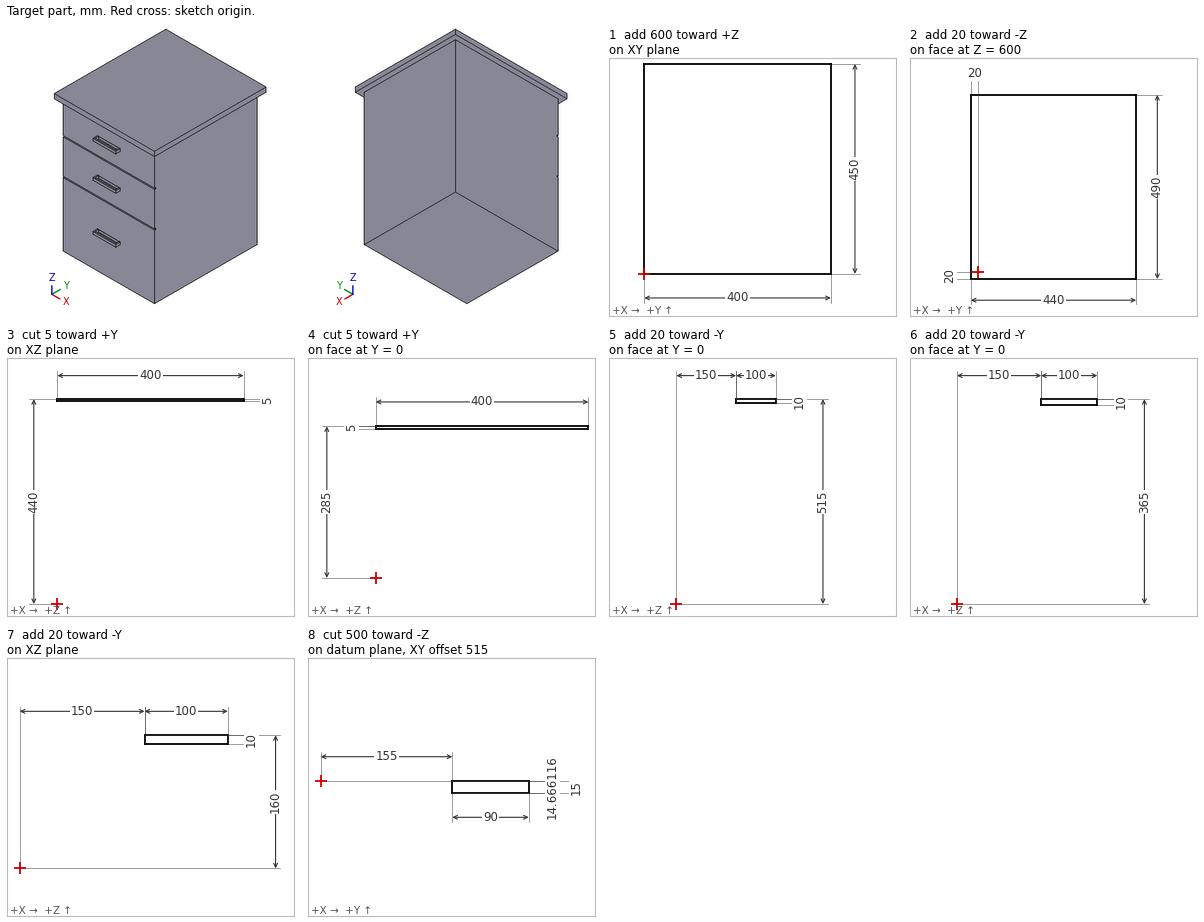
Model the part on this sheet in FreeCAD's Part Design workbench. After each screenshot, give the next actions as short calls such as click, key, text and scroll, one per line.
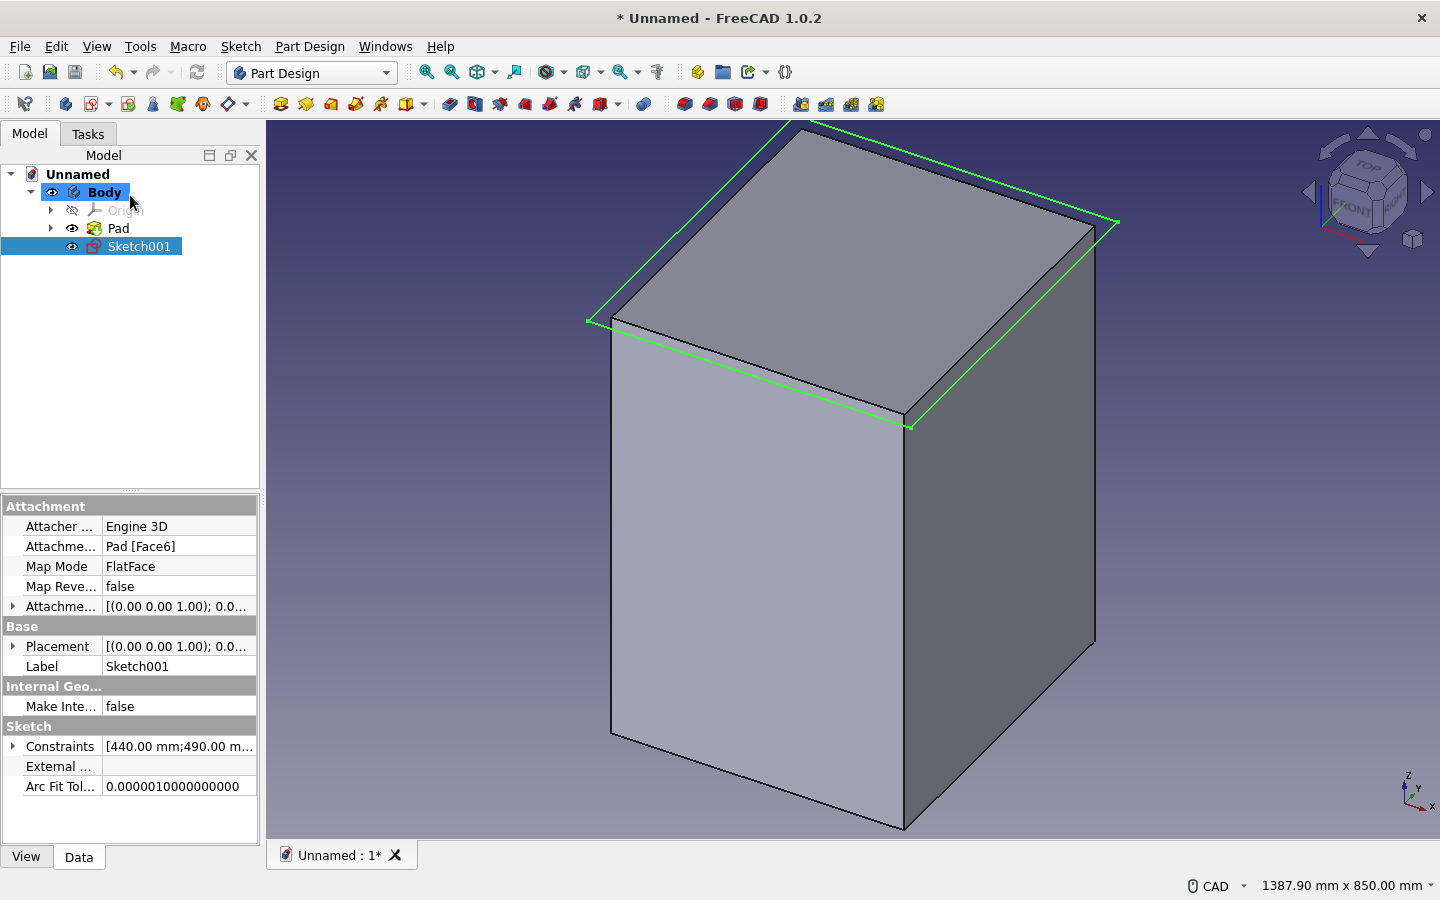
click(281, 104)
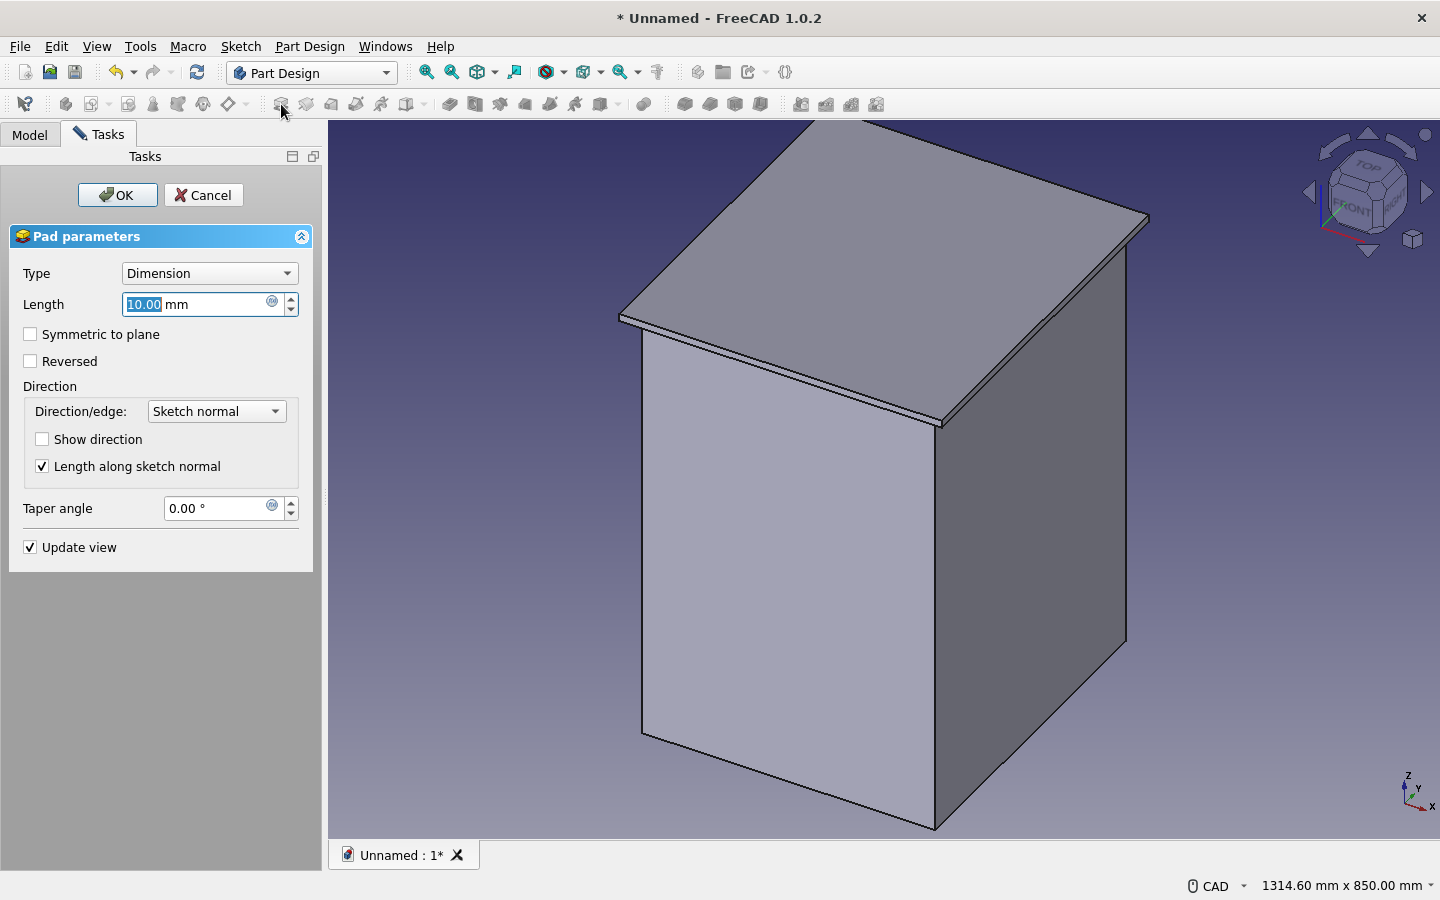
text(20)
key(Tab)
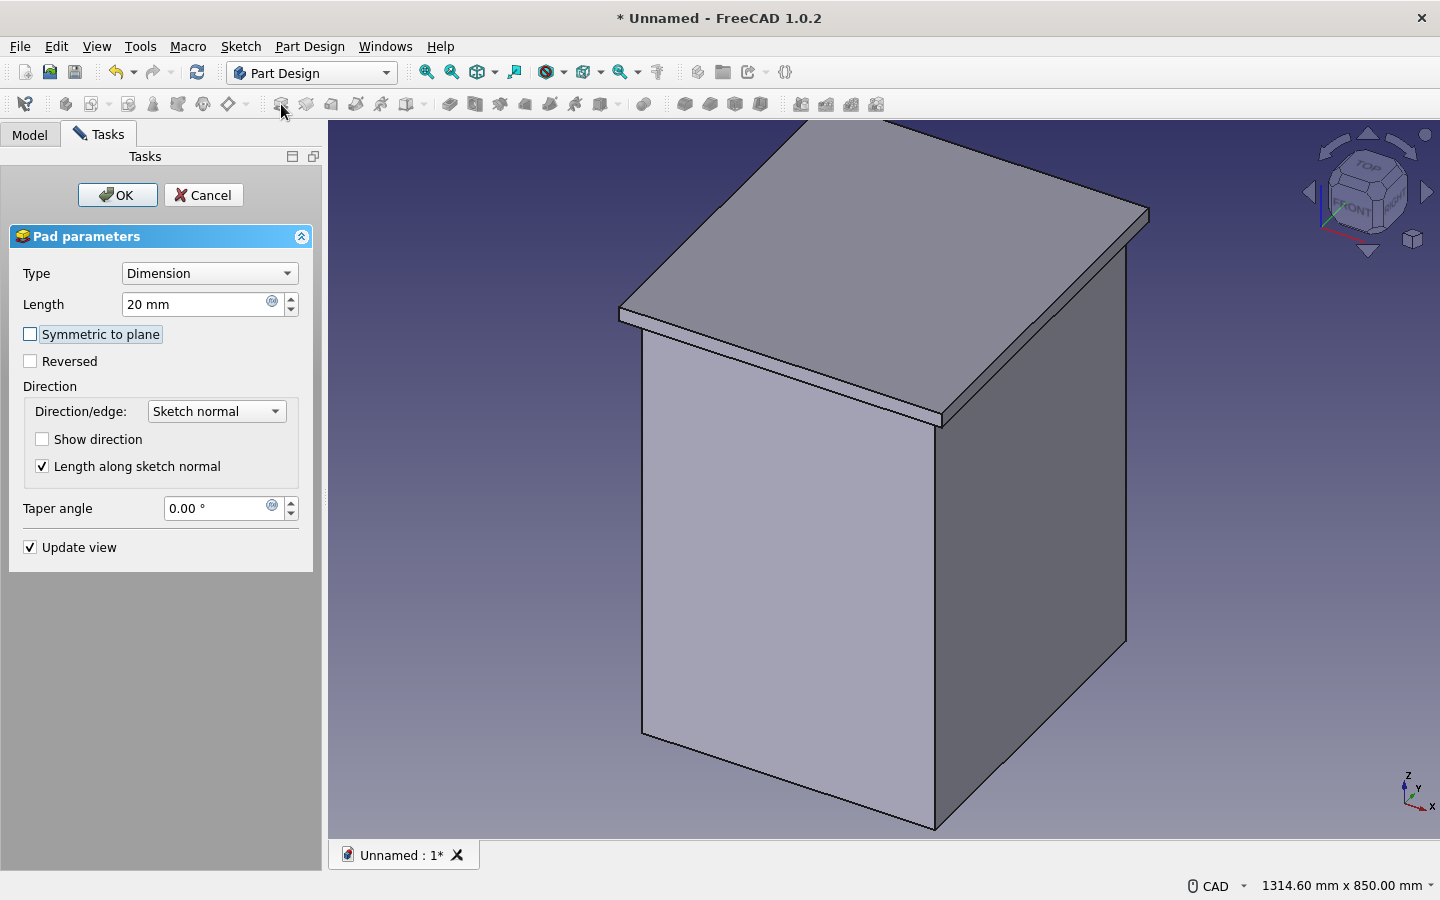
click(31, 361)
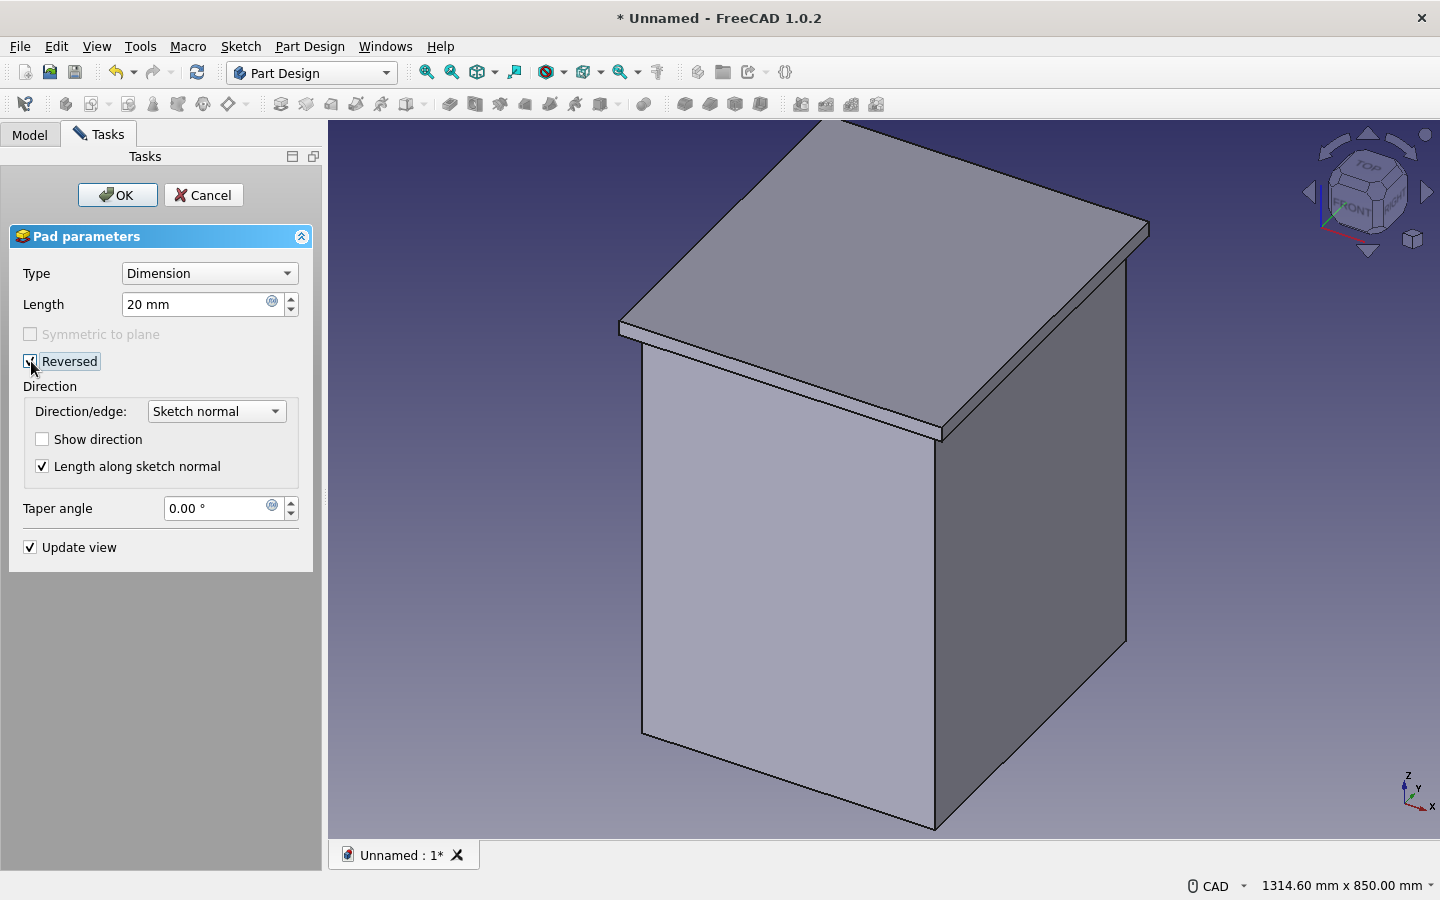
click(118, 195)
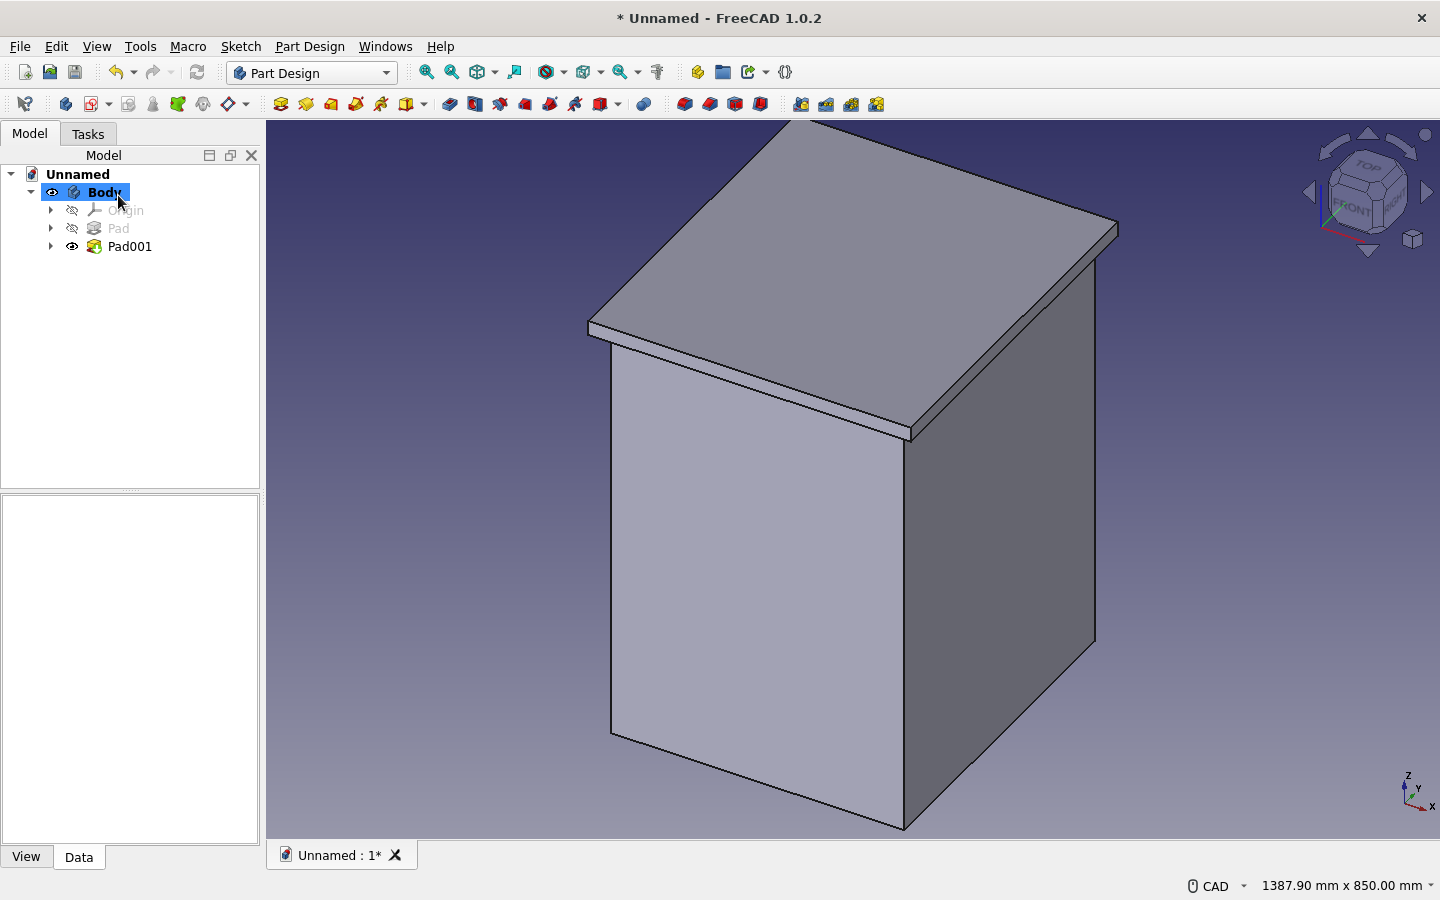
click(427, 72)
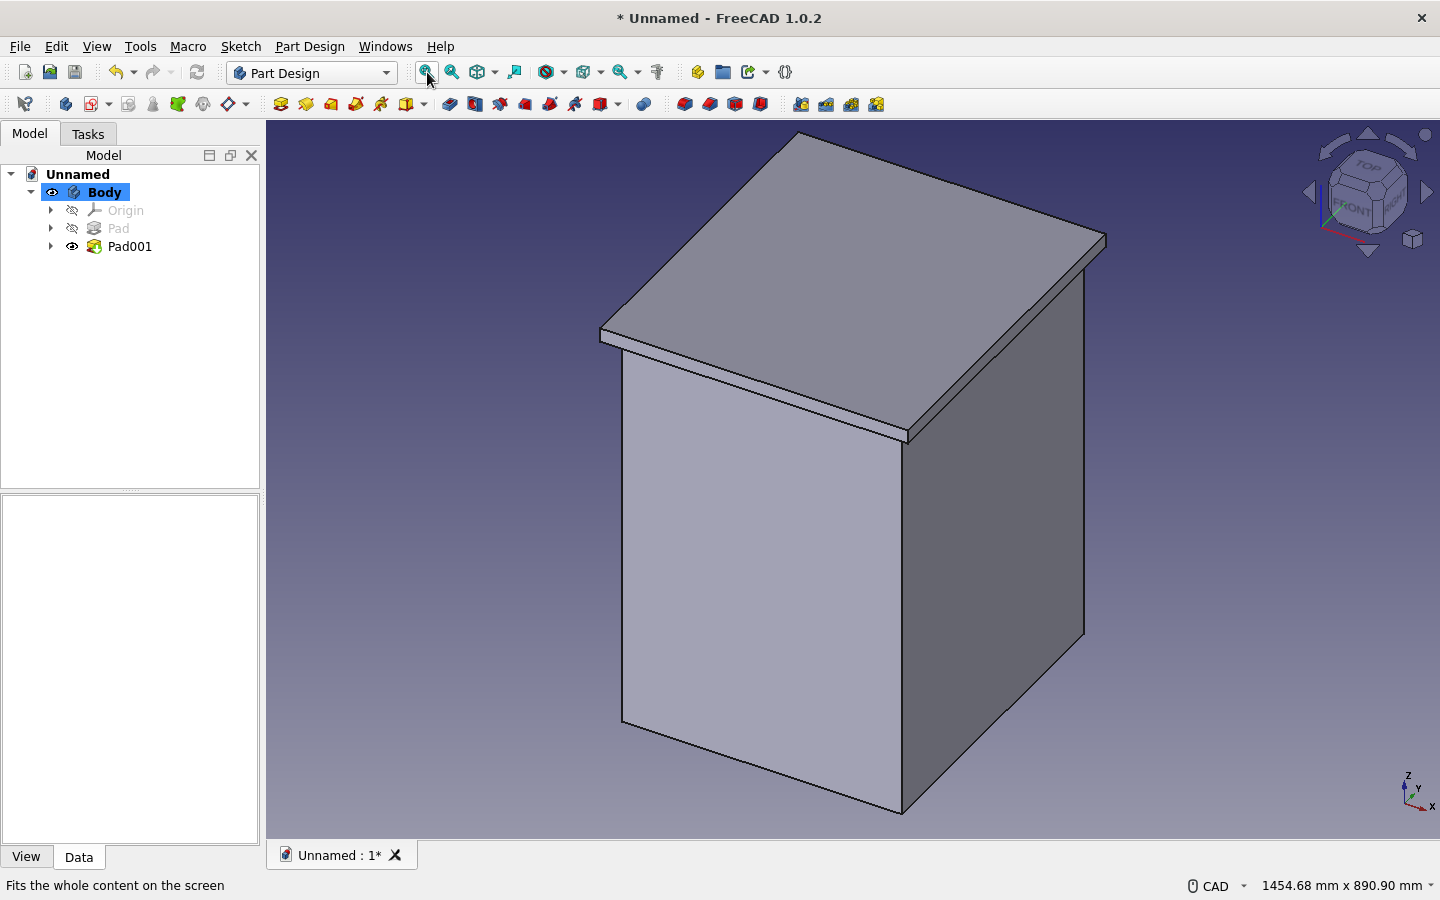
click(90, 104)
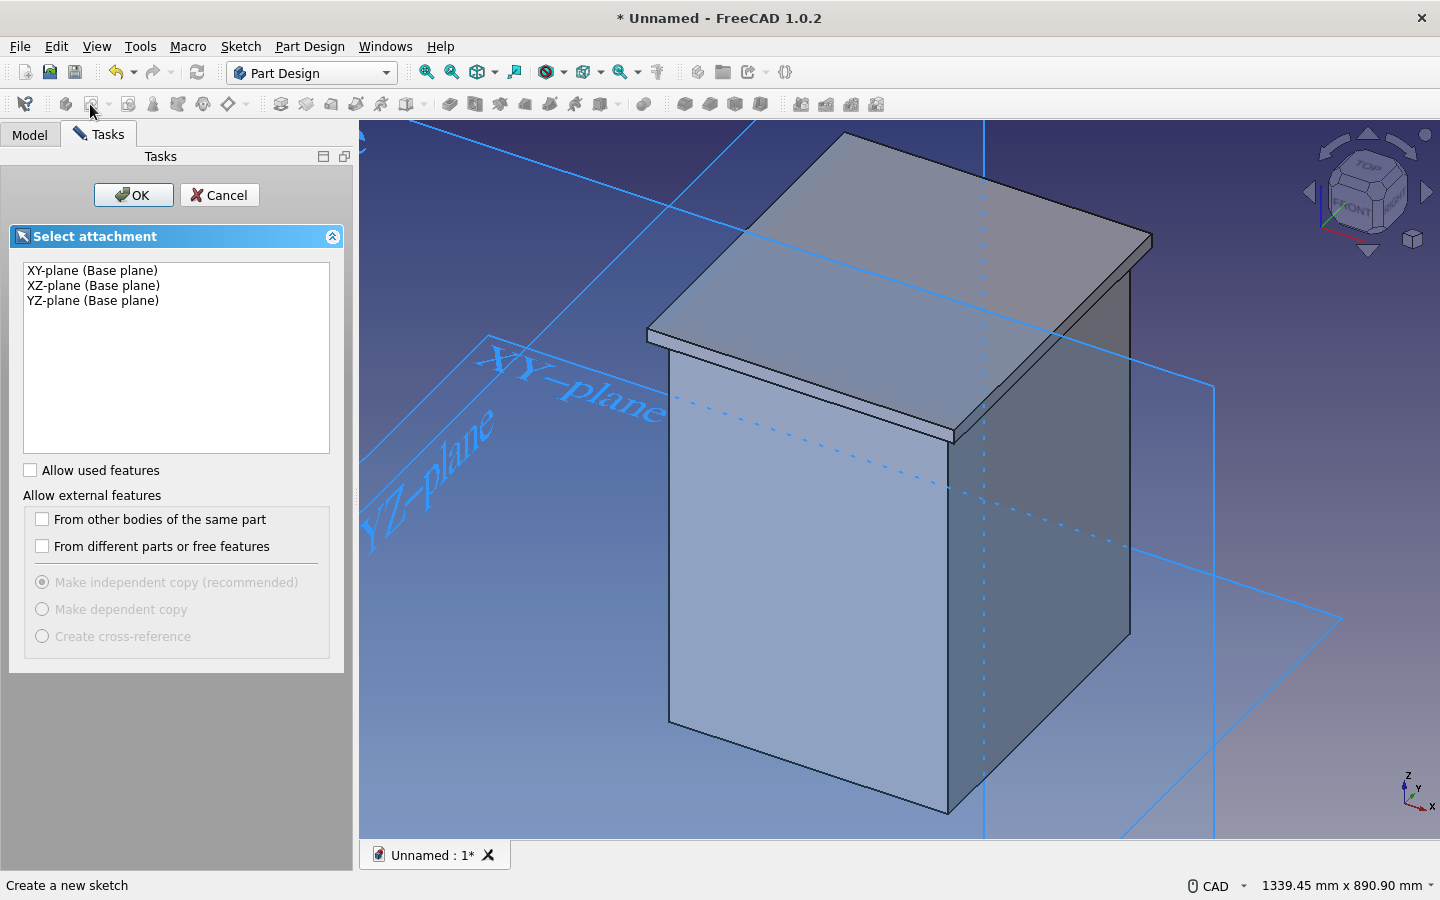
click(84, 286)